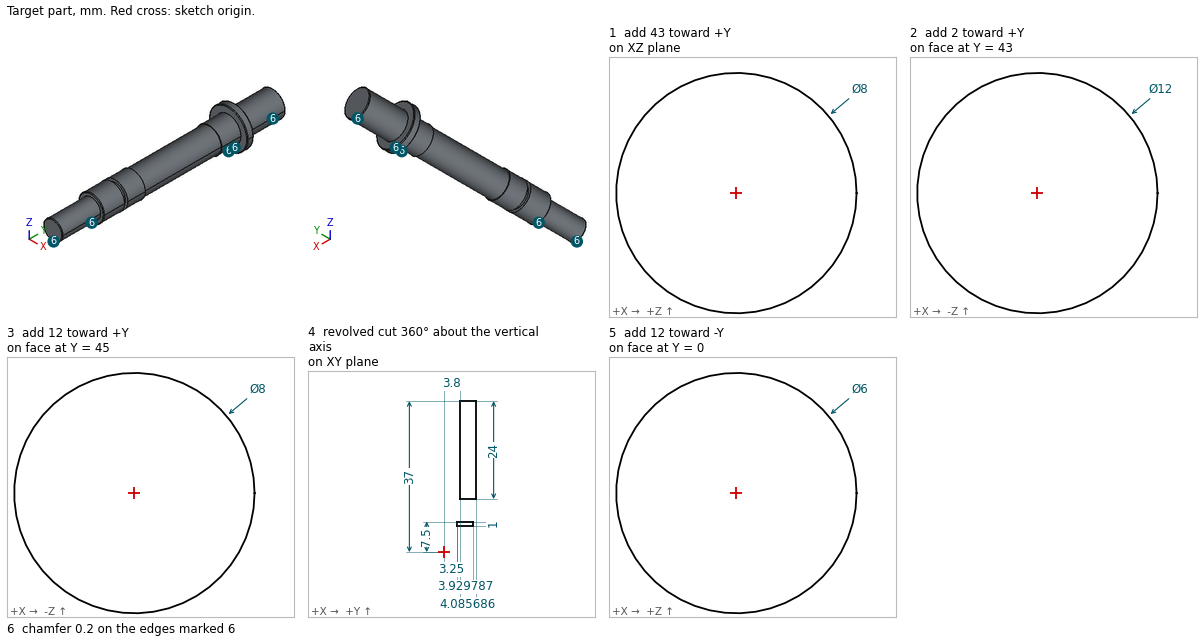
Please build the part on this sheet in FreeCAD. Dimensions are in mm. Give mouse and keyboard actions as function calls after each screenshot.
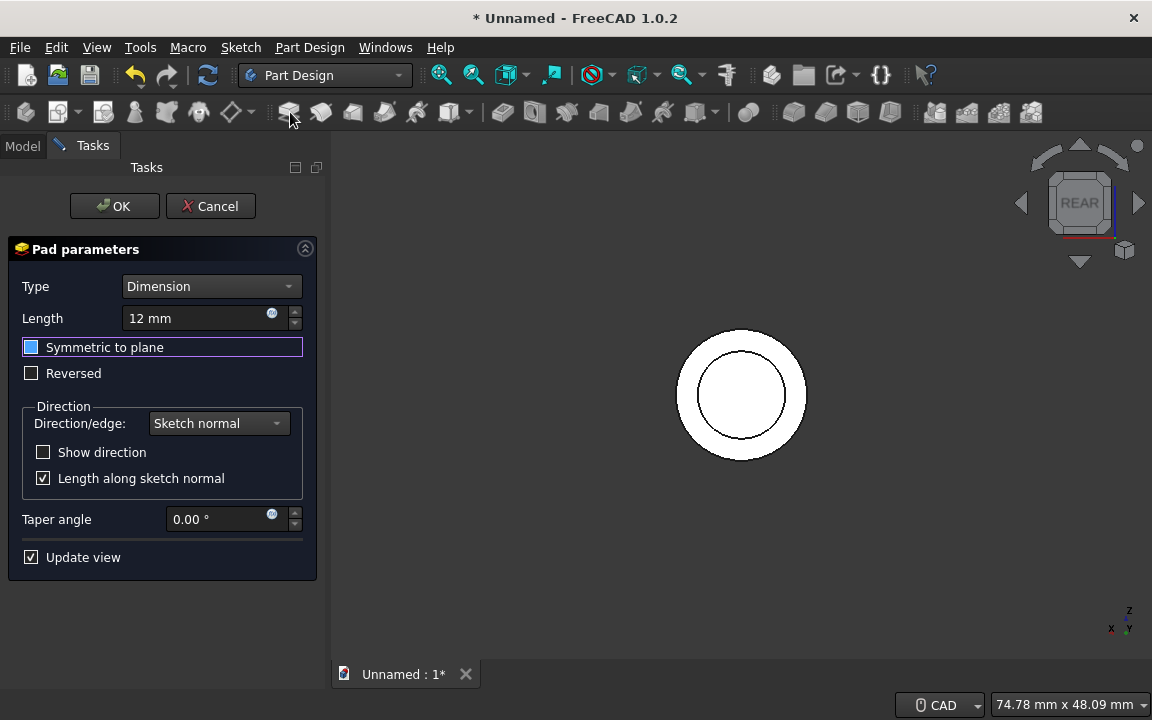
click(115, 206)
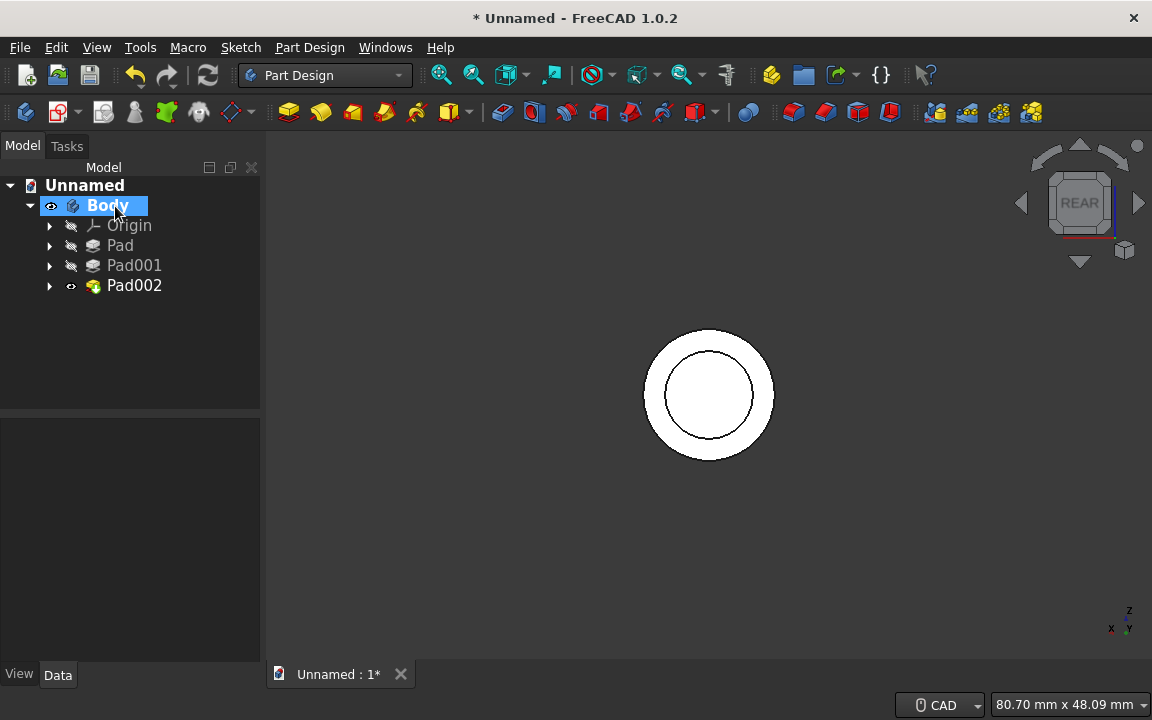
key(v)
key(f)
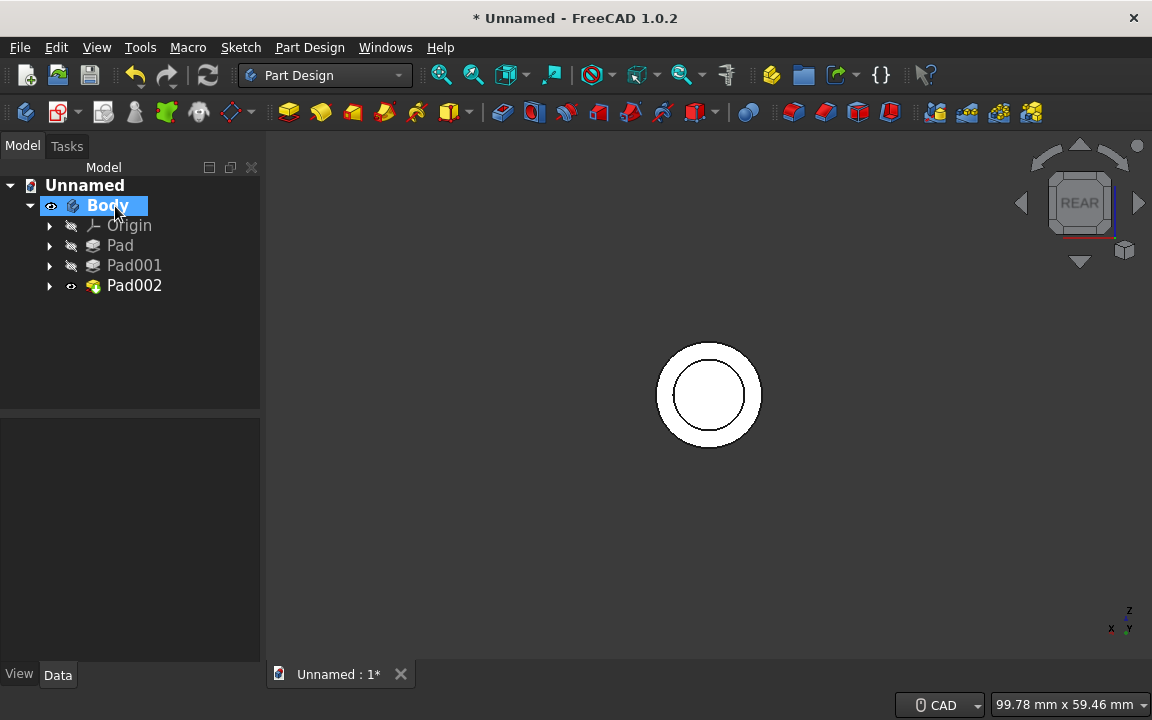
click(58, 112)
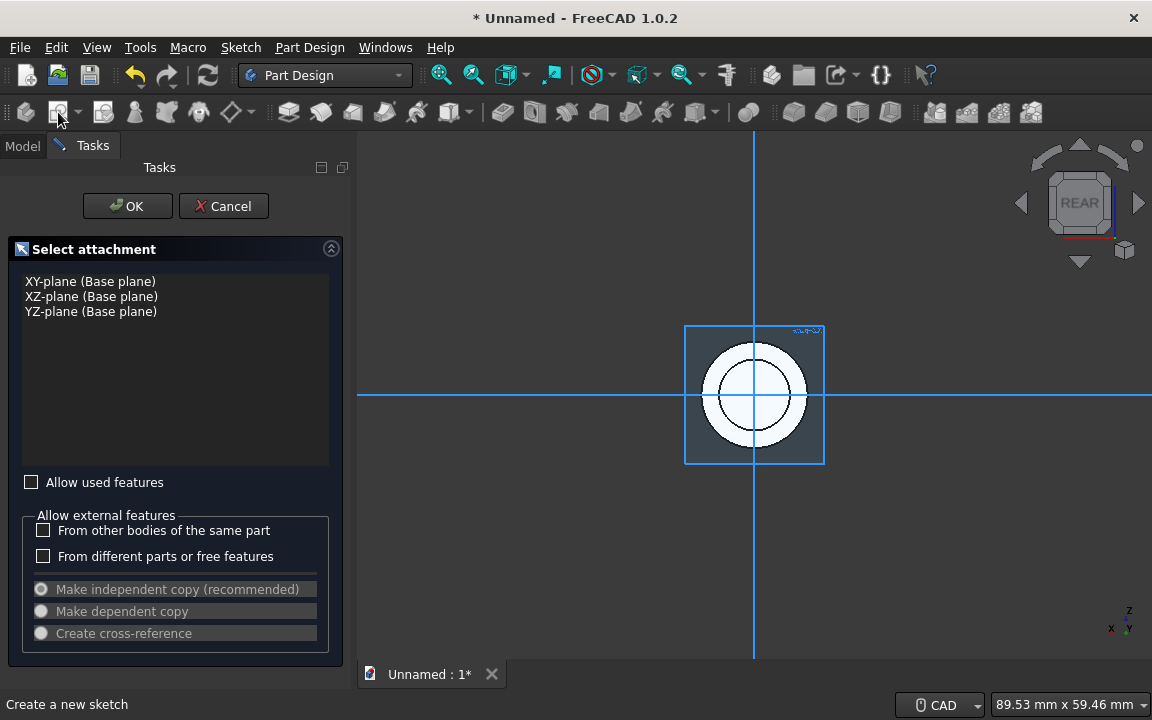
click(82, 282)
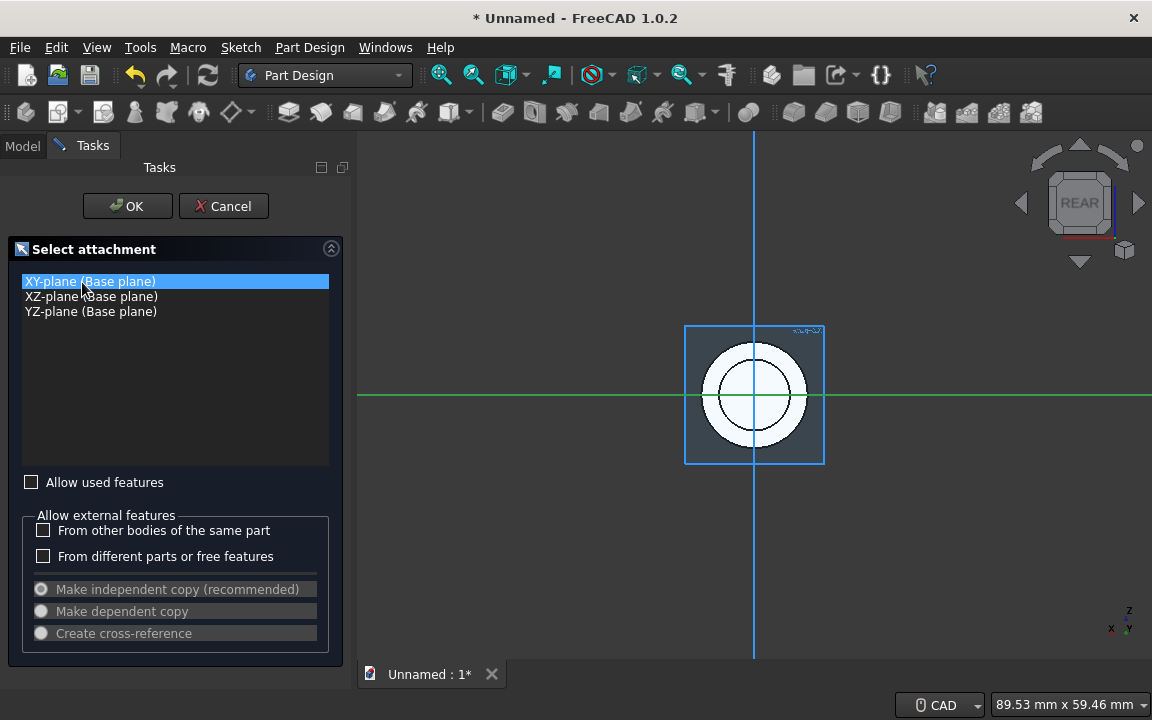
click(128, 206)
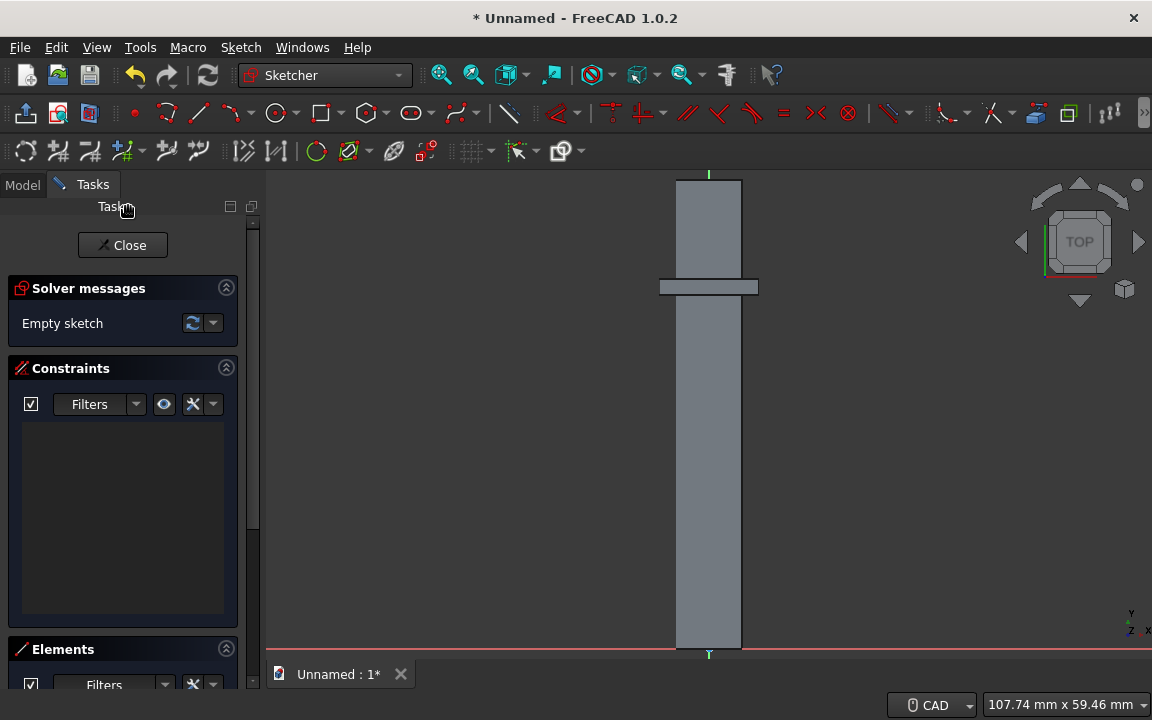
click(90, 114)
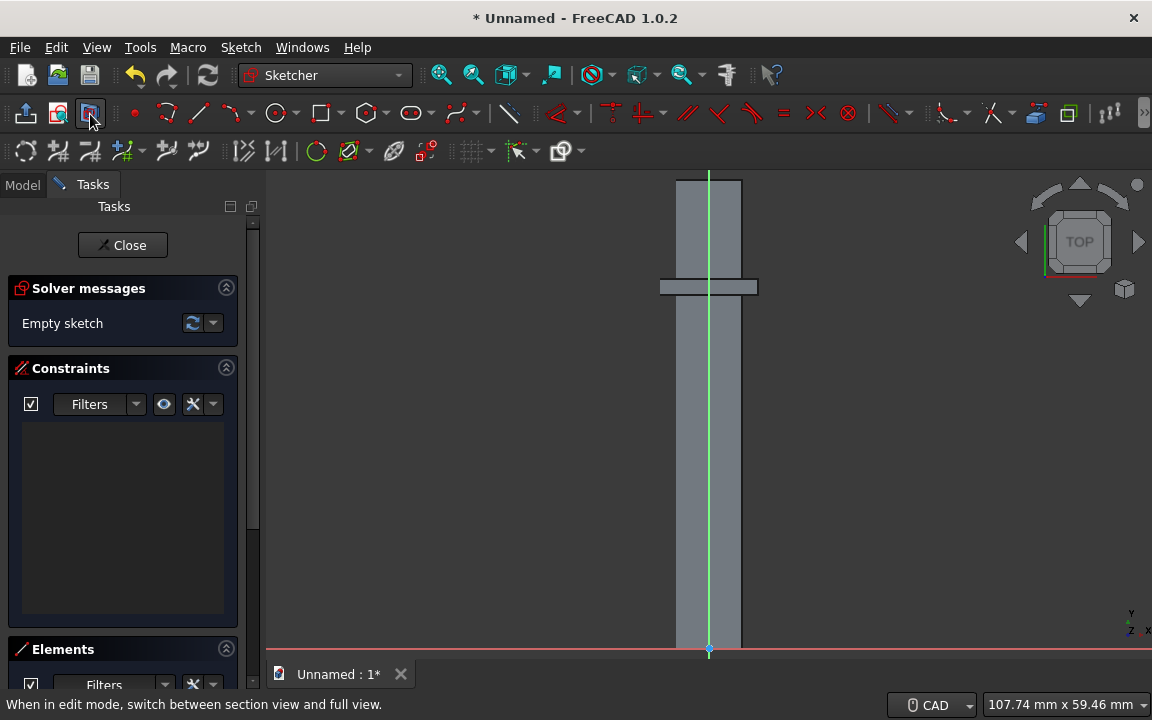
scroll(294, 198, down, 1)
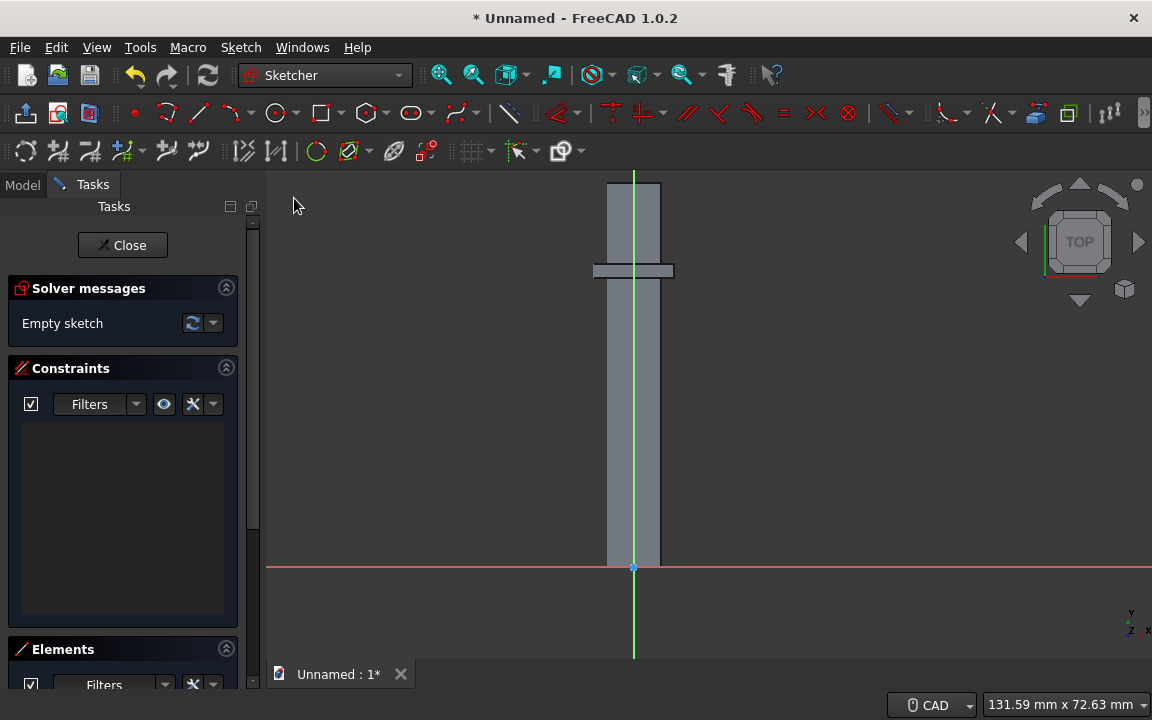
click(322, 114)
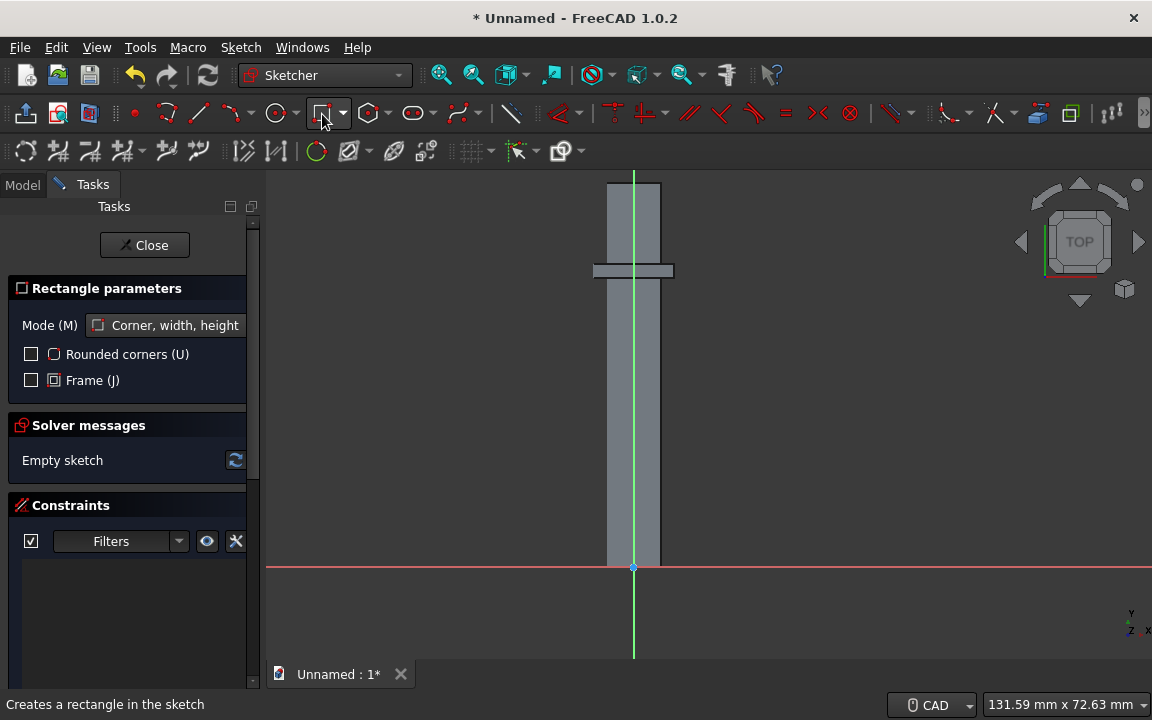
click(659, 318)
move(687, 480)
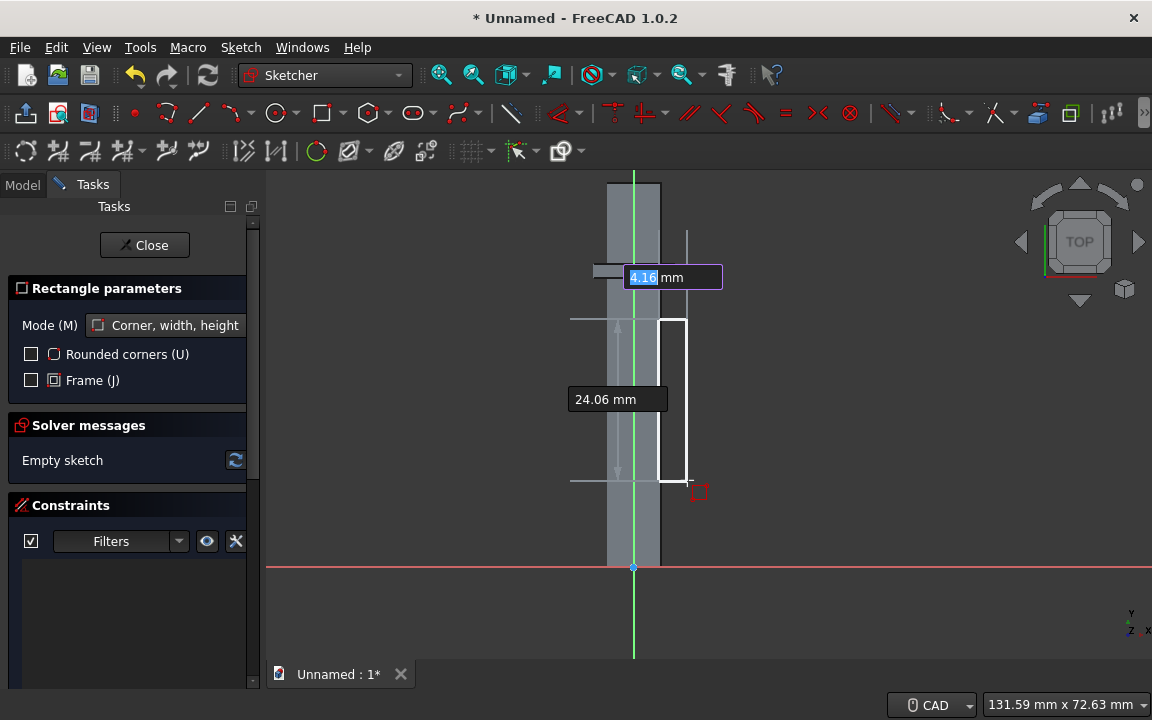
text(4.085686)
key(Tab)
text(24)
key(Return)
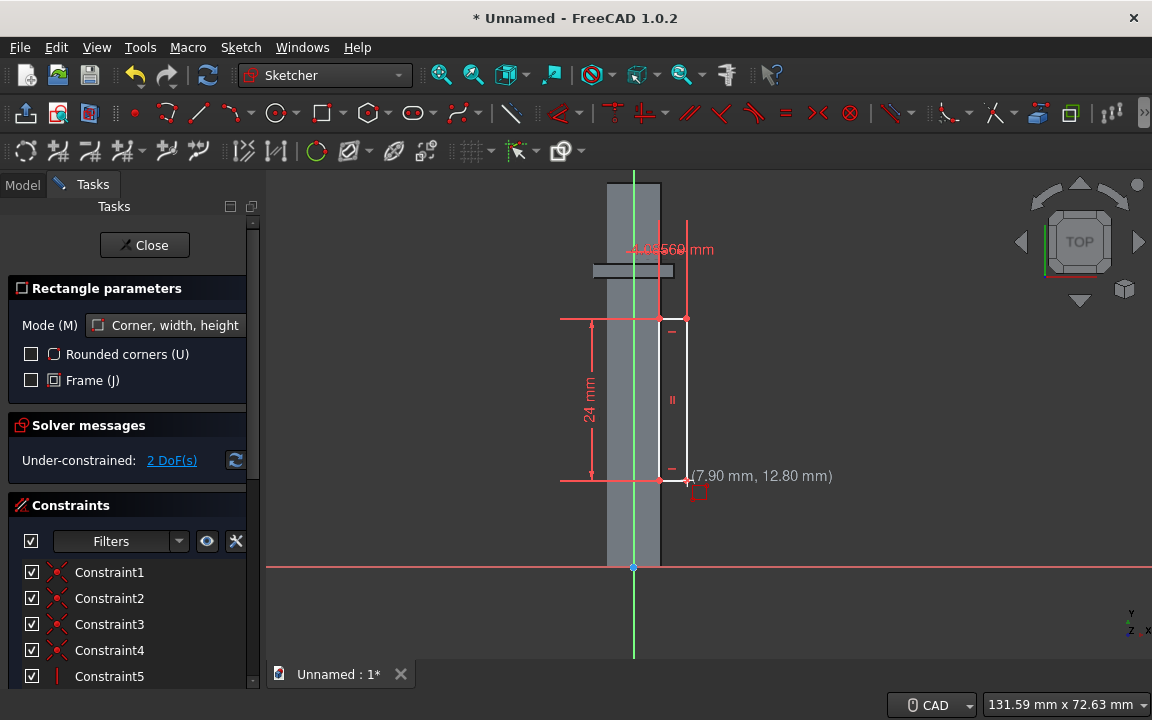
scroll(656, 517, up, 5)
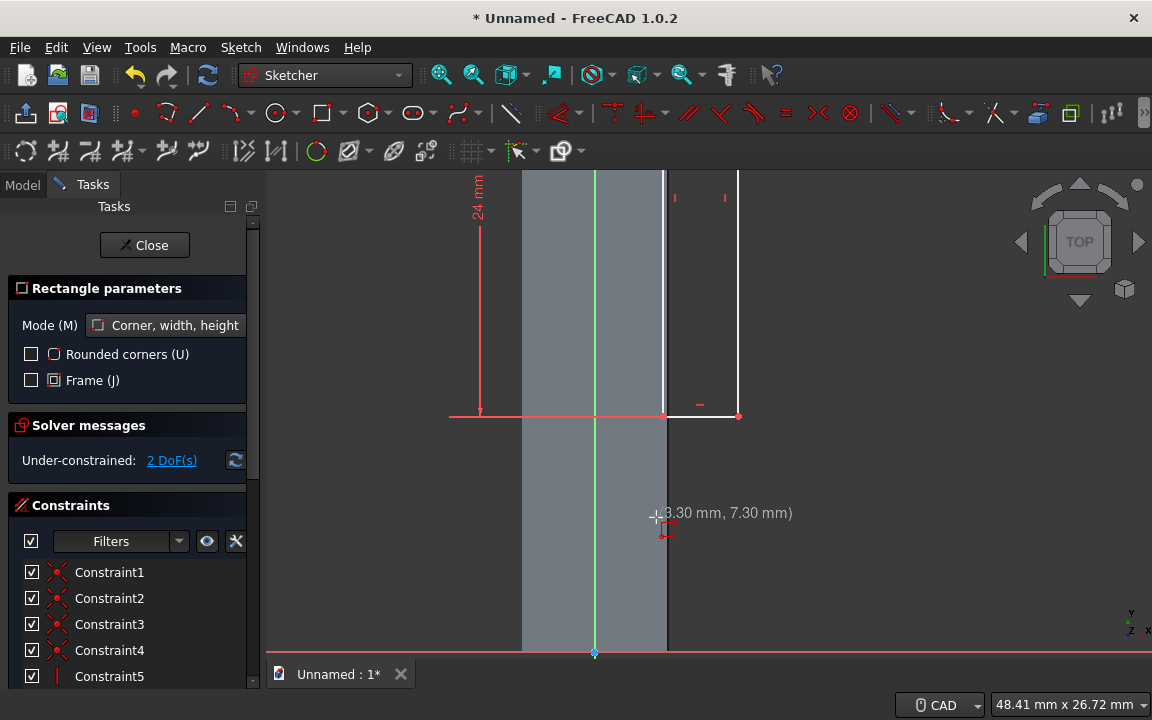
click(654, 515)
move(726, 533)